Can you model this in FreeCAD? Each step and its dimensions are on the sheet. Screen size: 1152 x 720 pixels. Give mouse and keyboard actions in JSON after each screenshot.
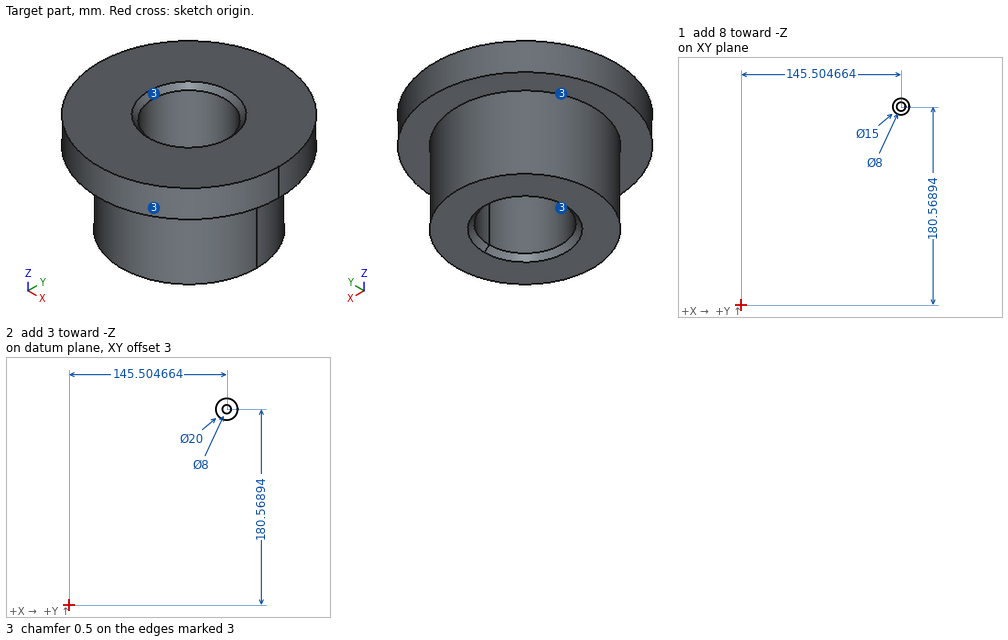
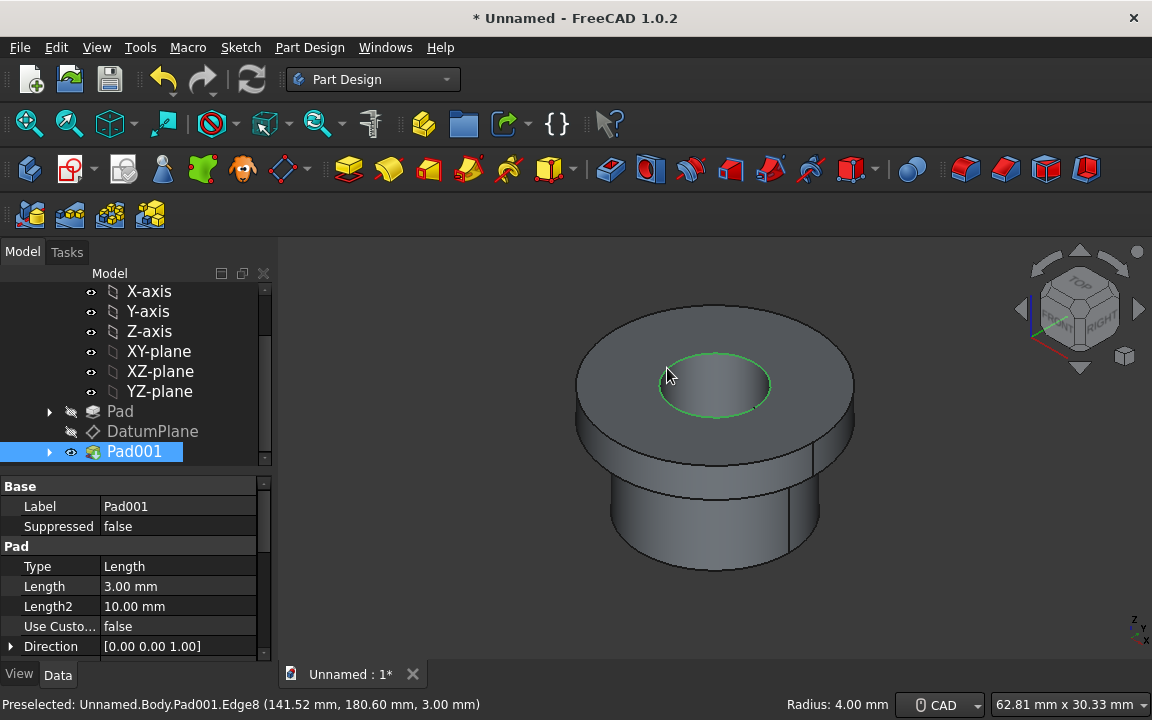
{"action": "key", "text": "2"}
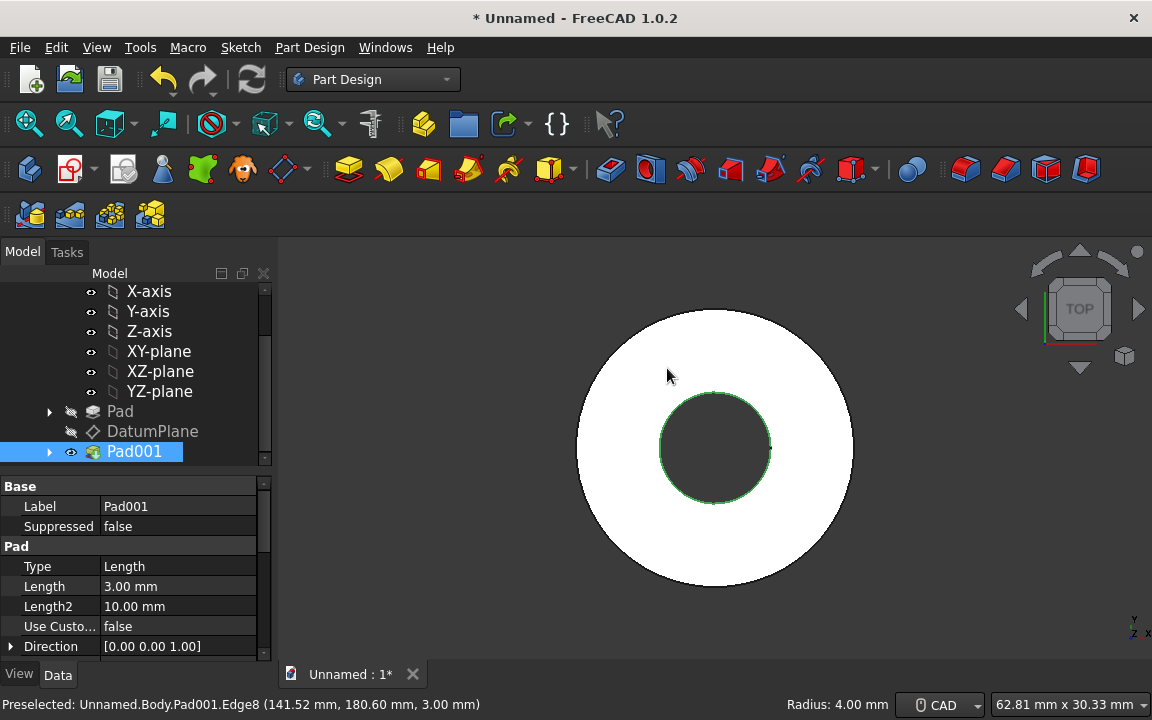
{"action": "key", "text": "1"}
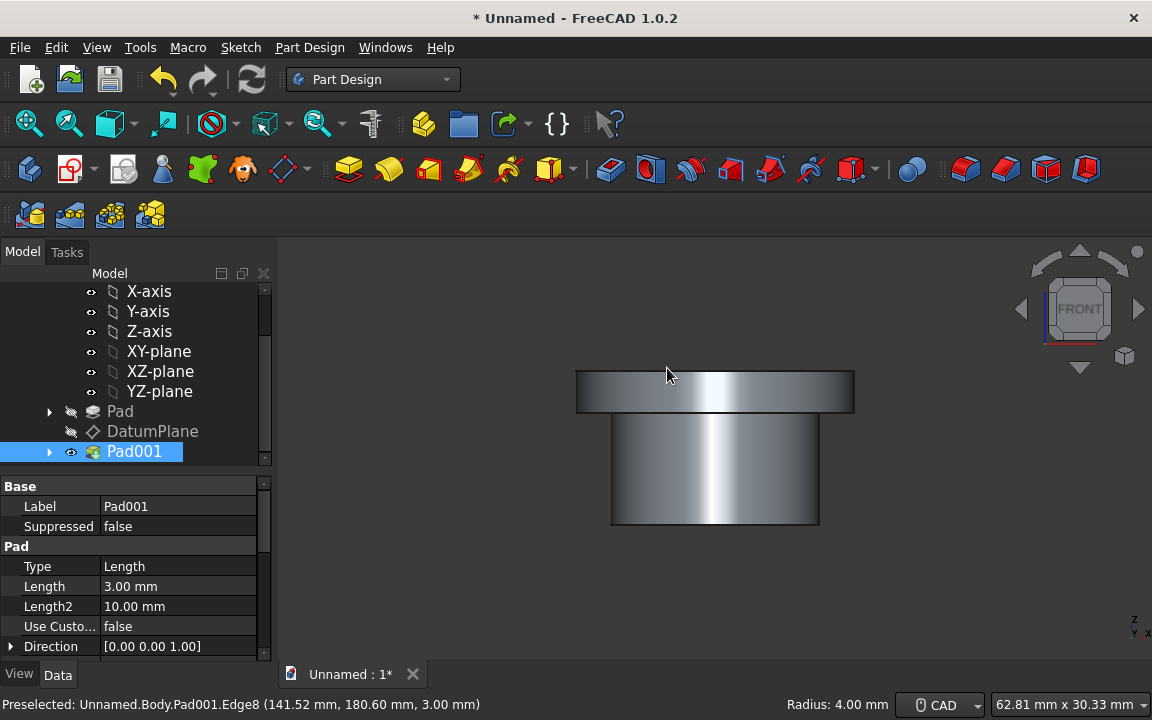
{"action": "left_click", "coordinate": [30, 124]}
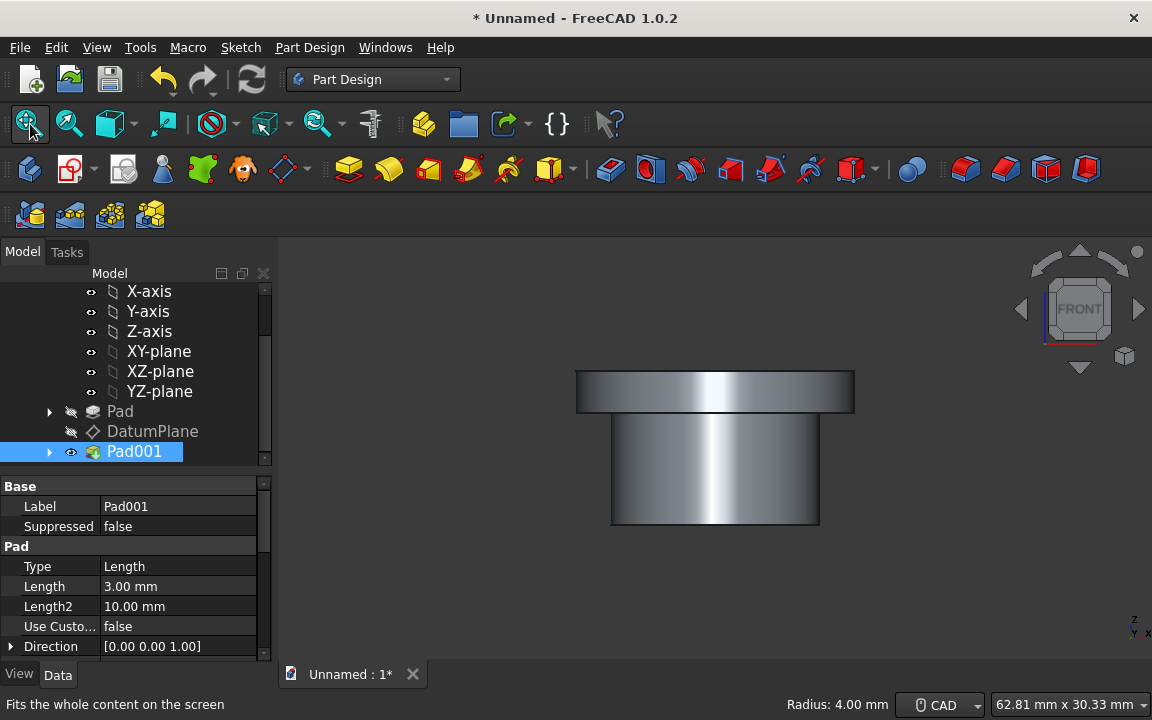
{"action": "key", "text": "3"}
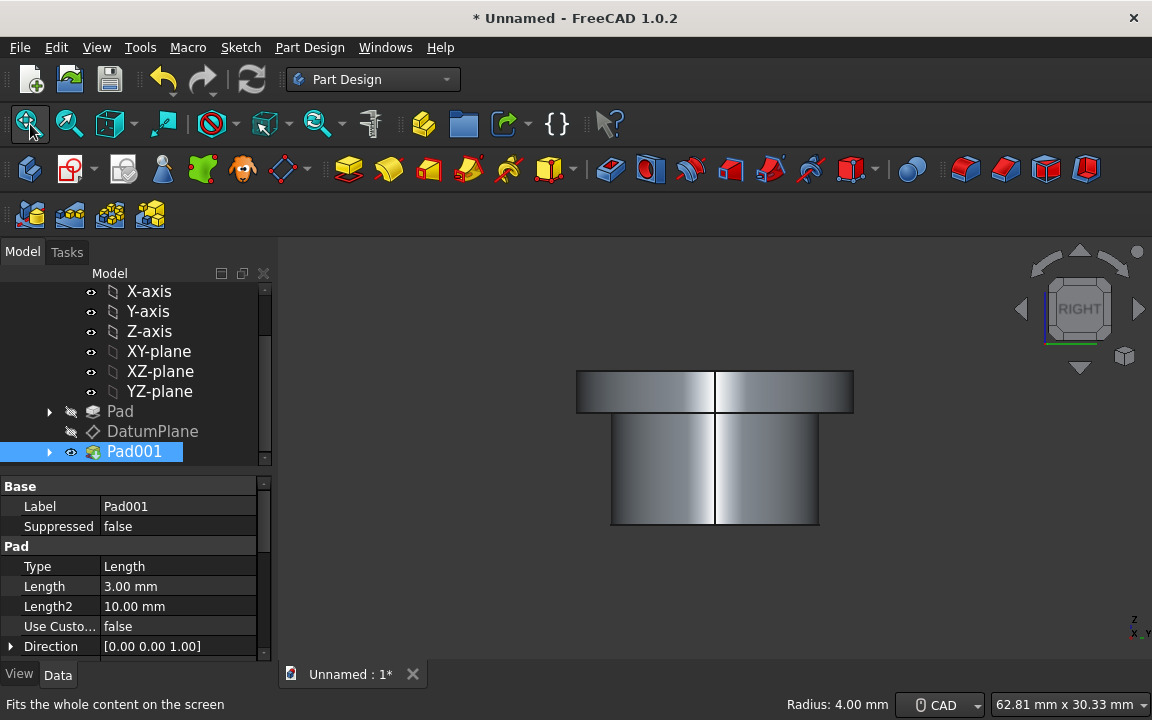
{"action": "left_click", "coordinate": [30, 124]}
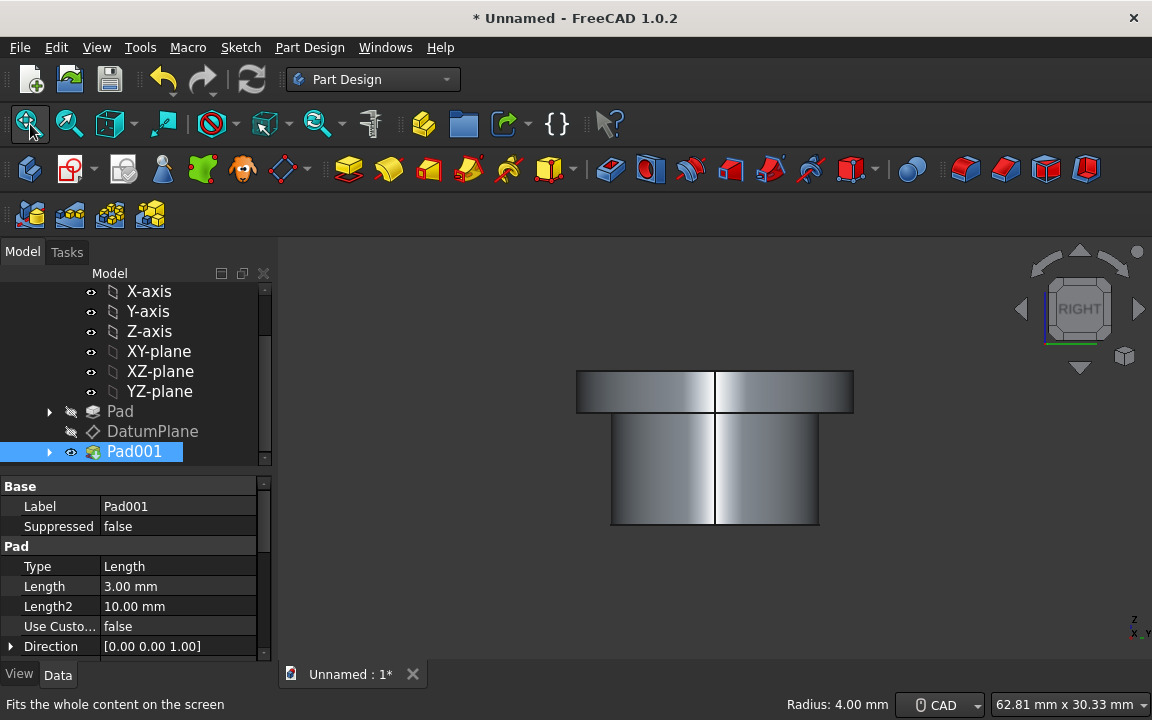
{"action": "key", "text": "5"}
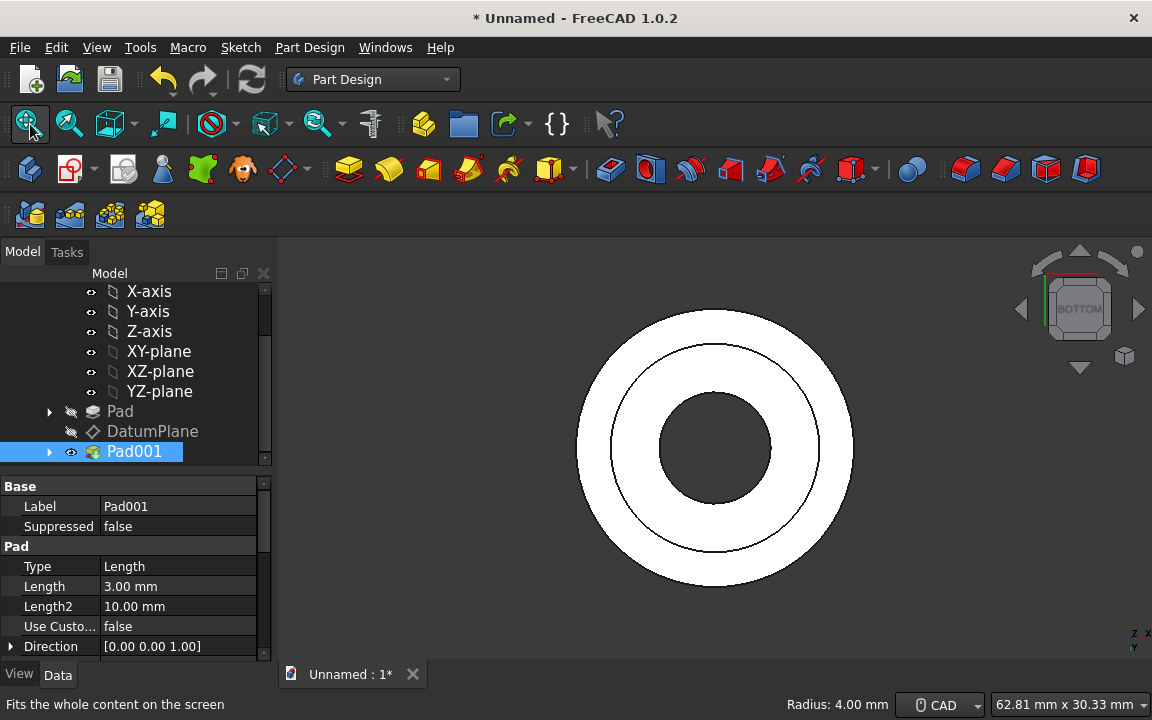
{"action": "left_click", "coordinate": [659, 447], "text": "ctrl"}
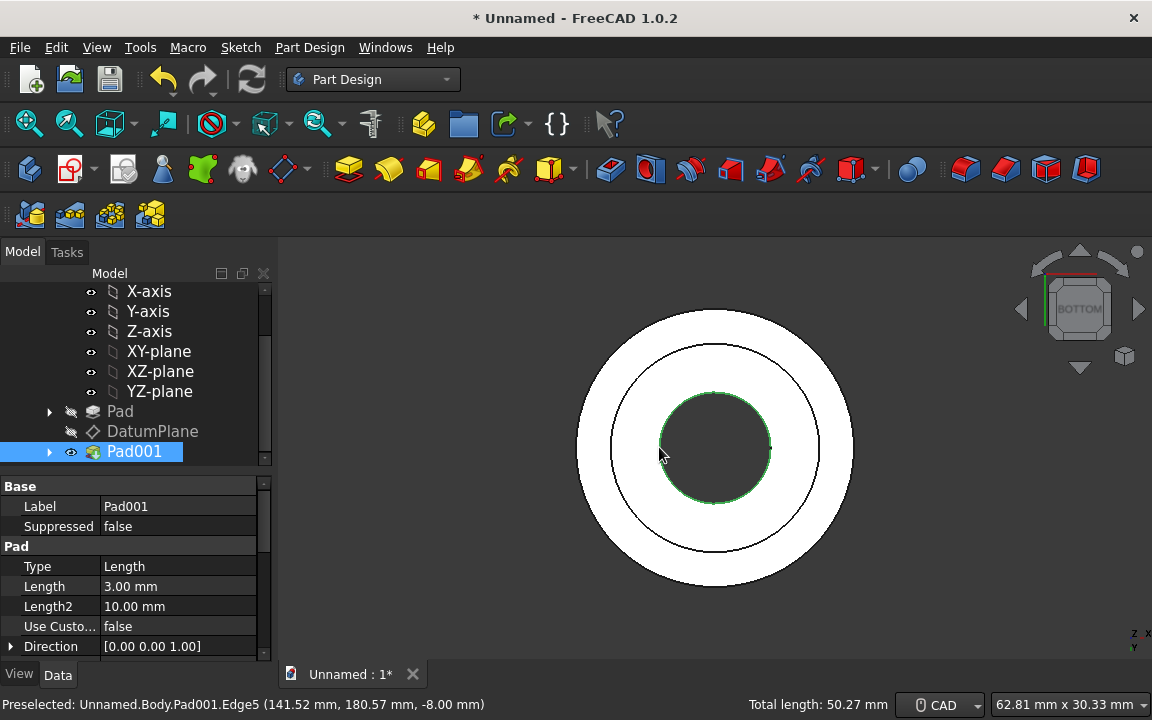
{"action": "left_click", "coordinate": [1006, 170]}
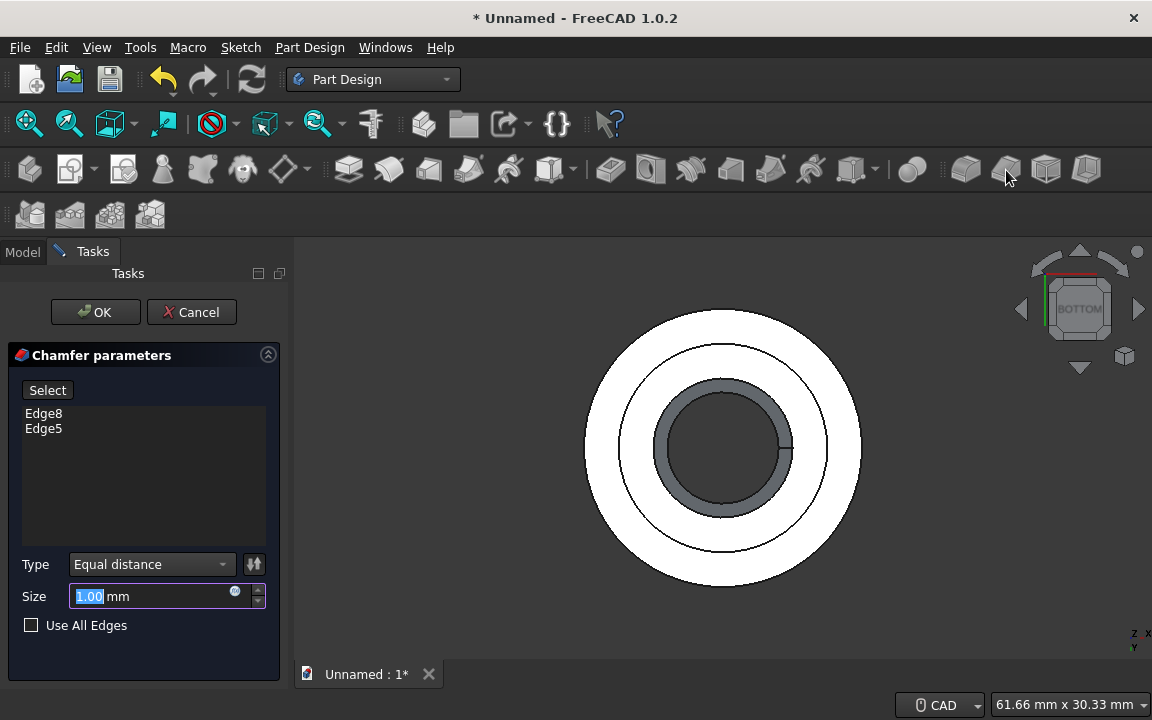
{"action": "type", "text": "0.5"}
{"action": "key", "text": "Tab"}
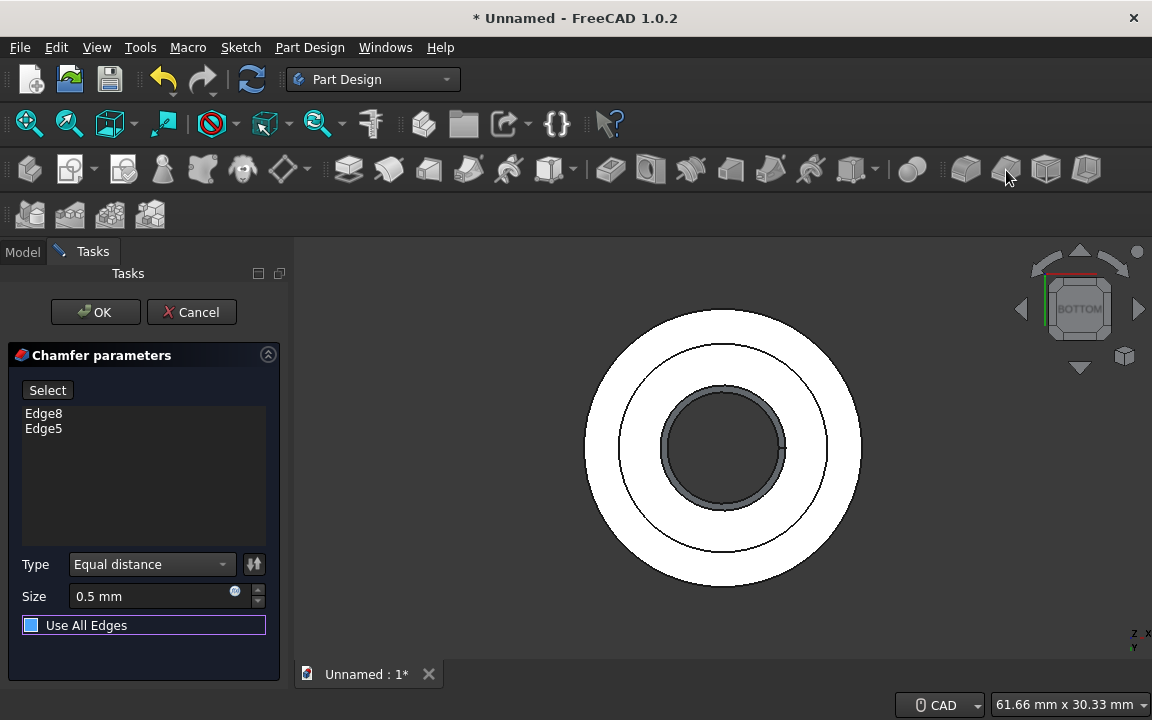
{"action": "left_click", "coordinate": [96, 312]}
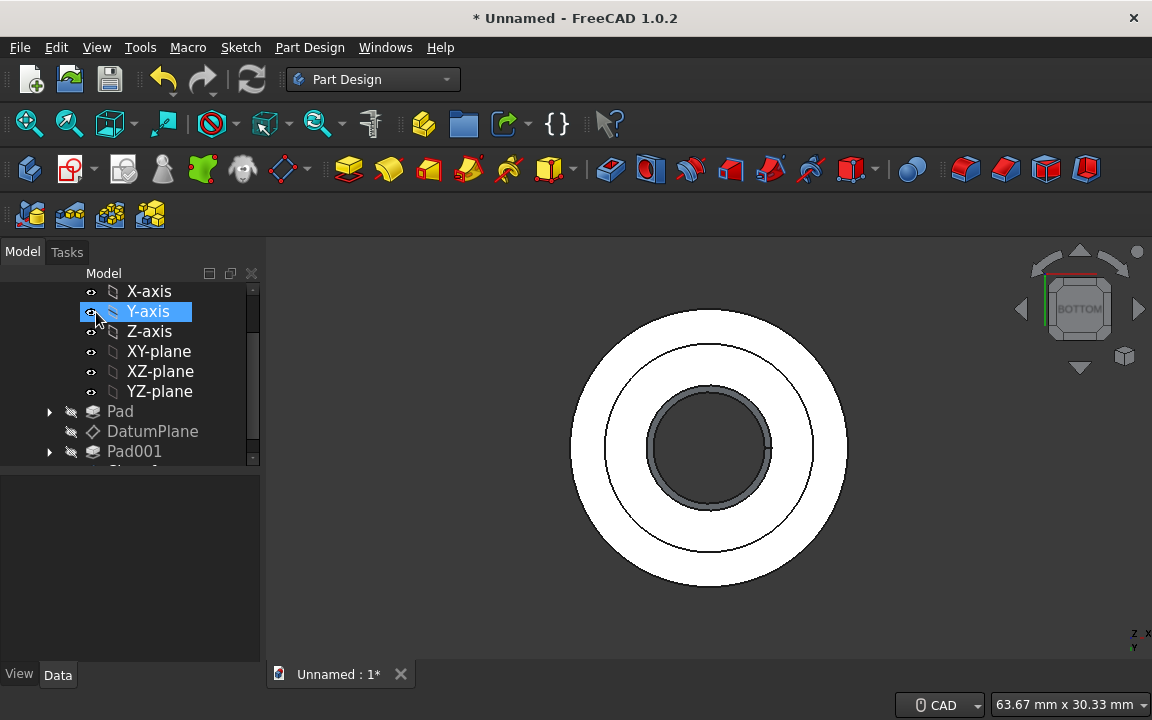
{"action": "key", "text": "0"}